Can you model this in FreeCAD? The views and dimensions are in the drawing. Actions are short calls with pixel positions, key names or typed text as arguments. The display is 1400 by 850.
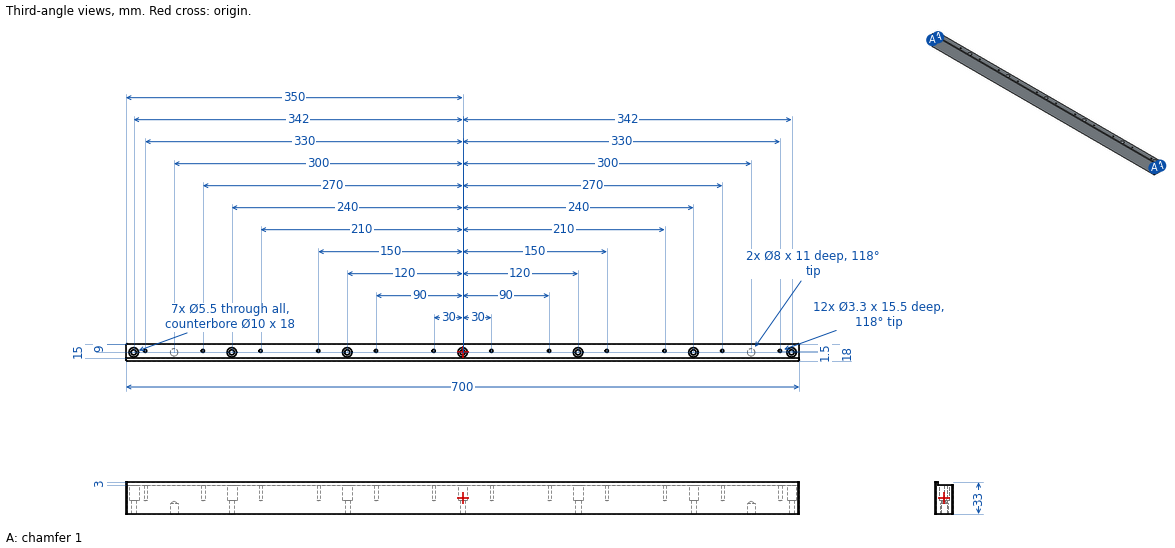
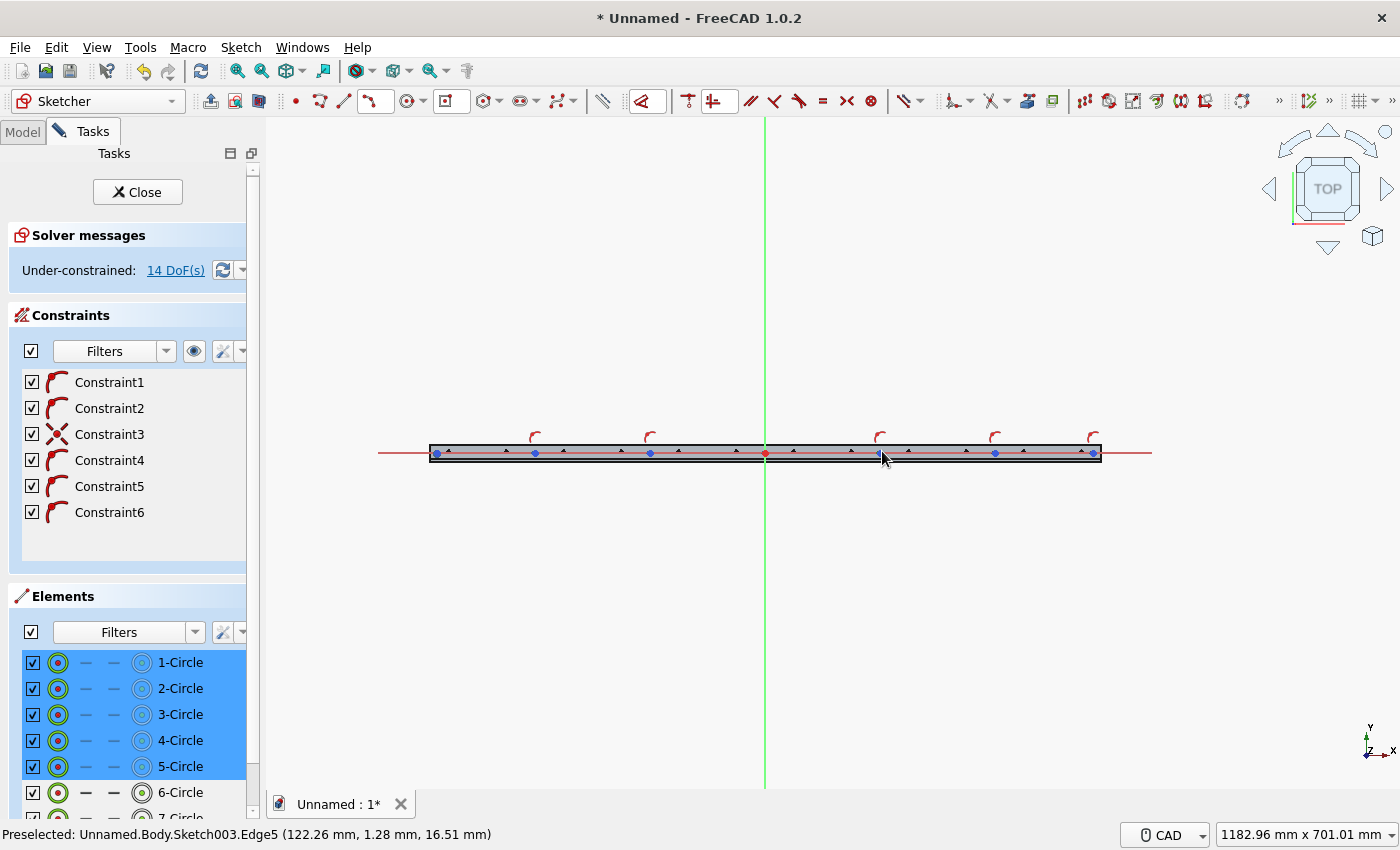
scroll(997, 451, up, 11)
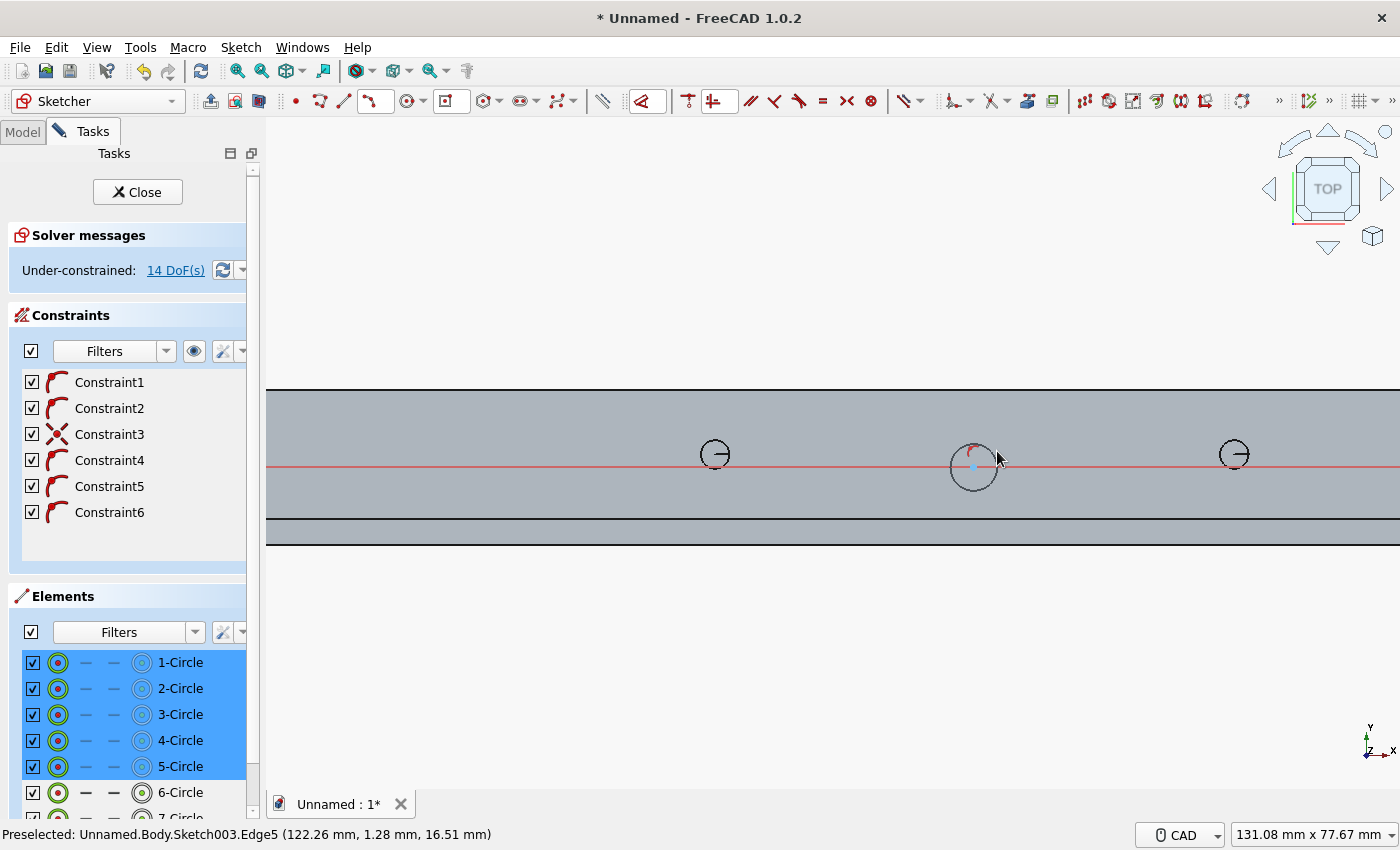
click(990, 451)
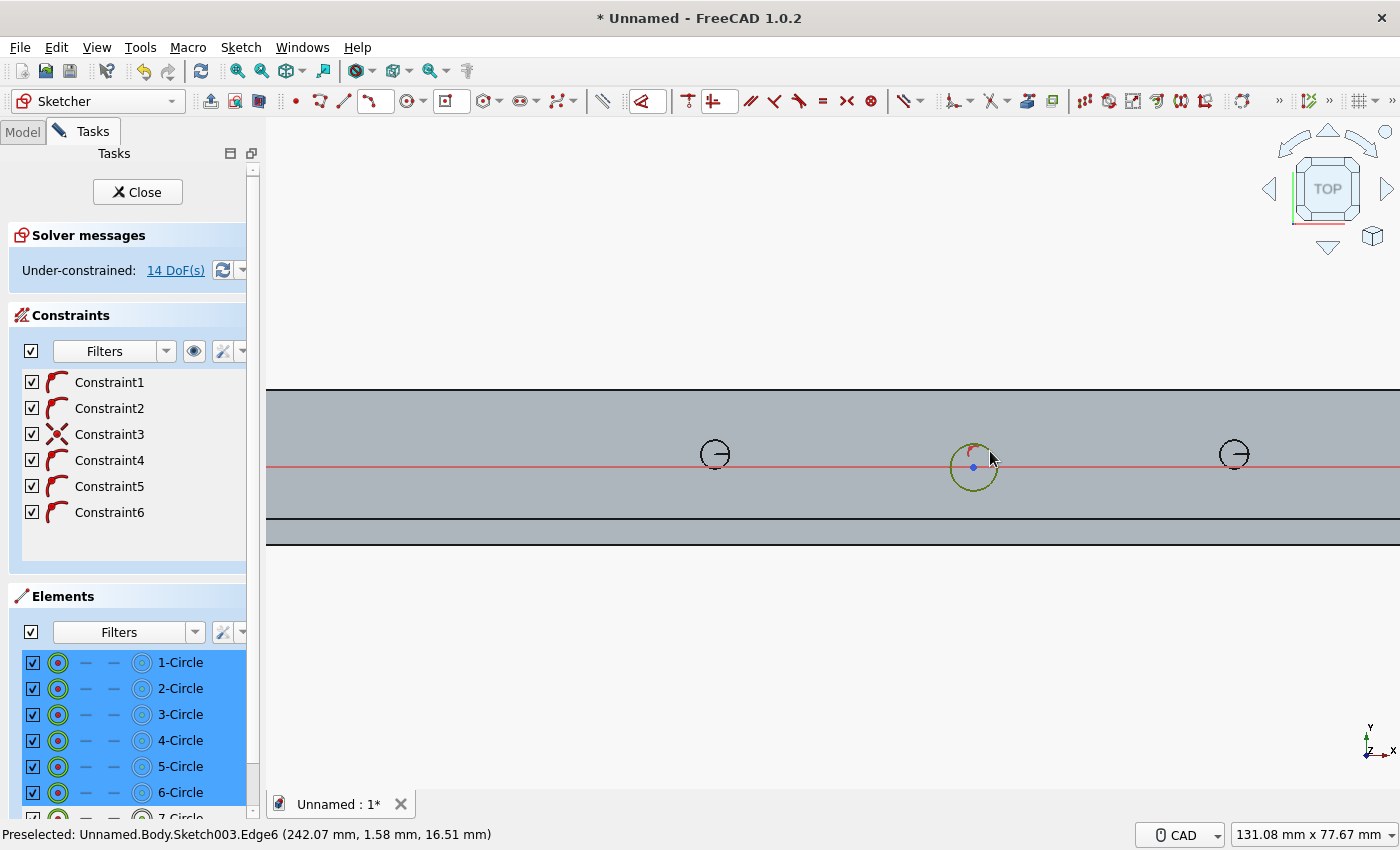
scroll(997, 451, down, 11)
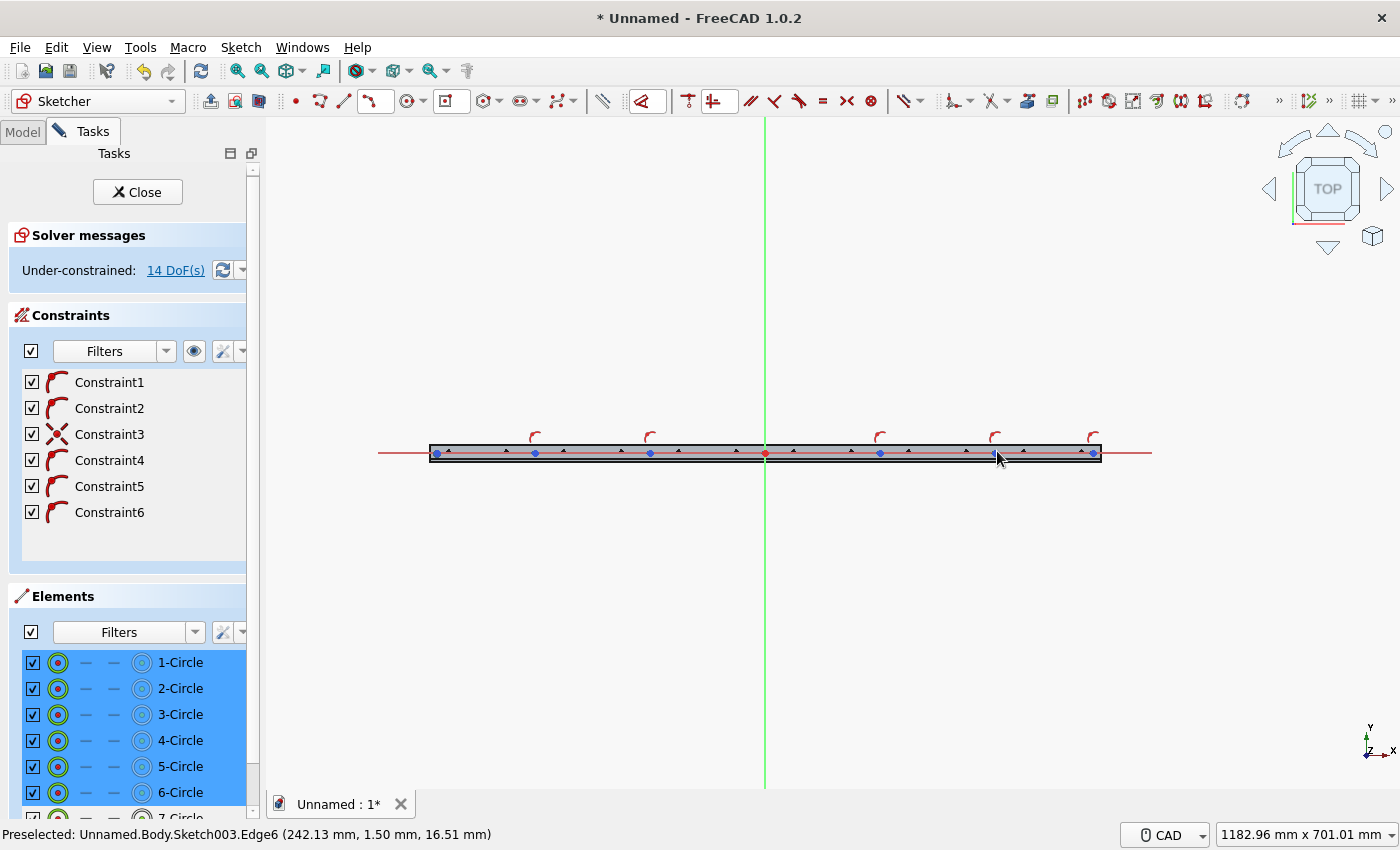
scroll(1095, 451, up, 11)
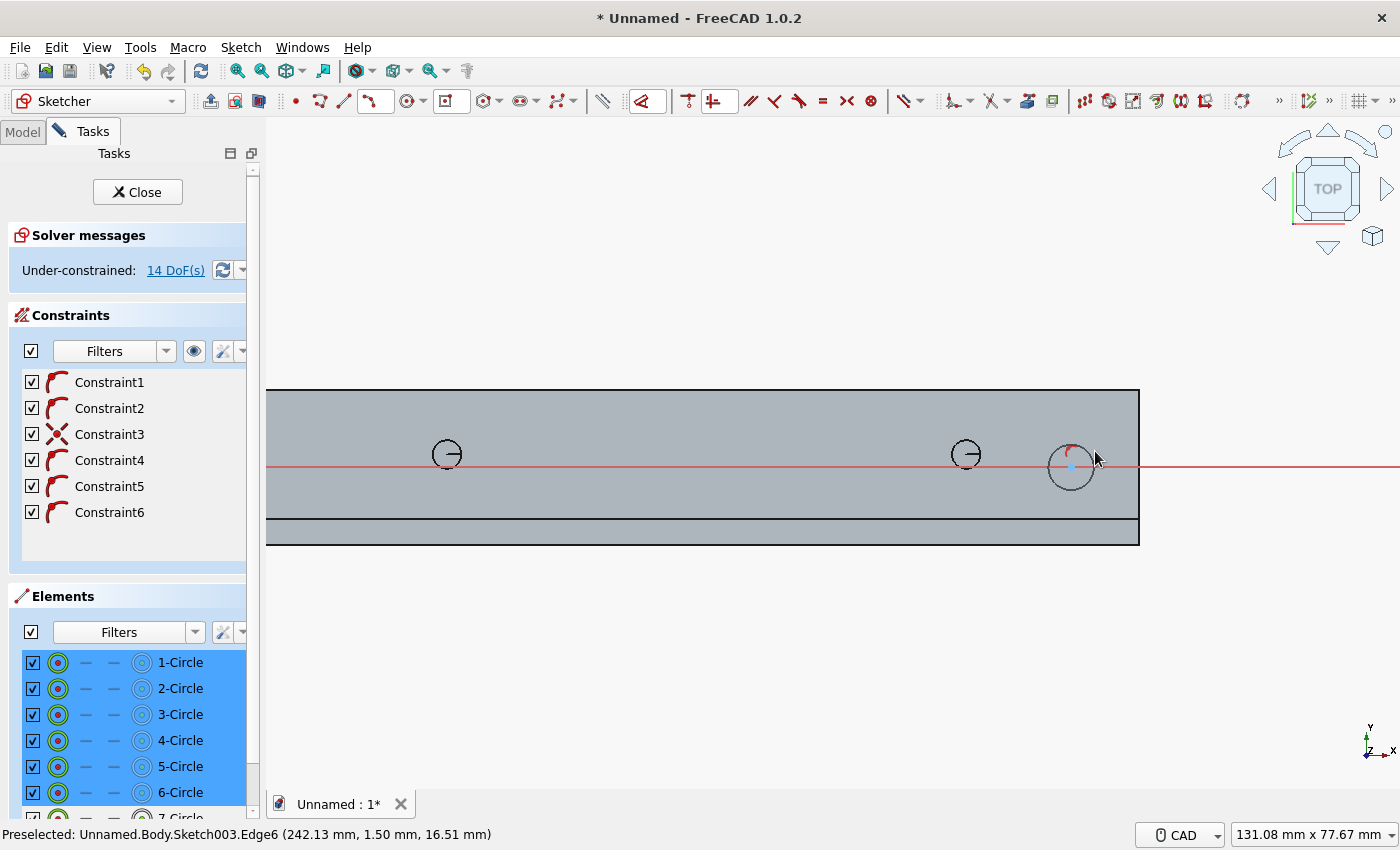
click(1087, 451)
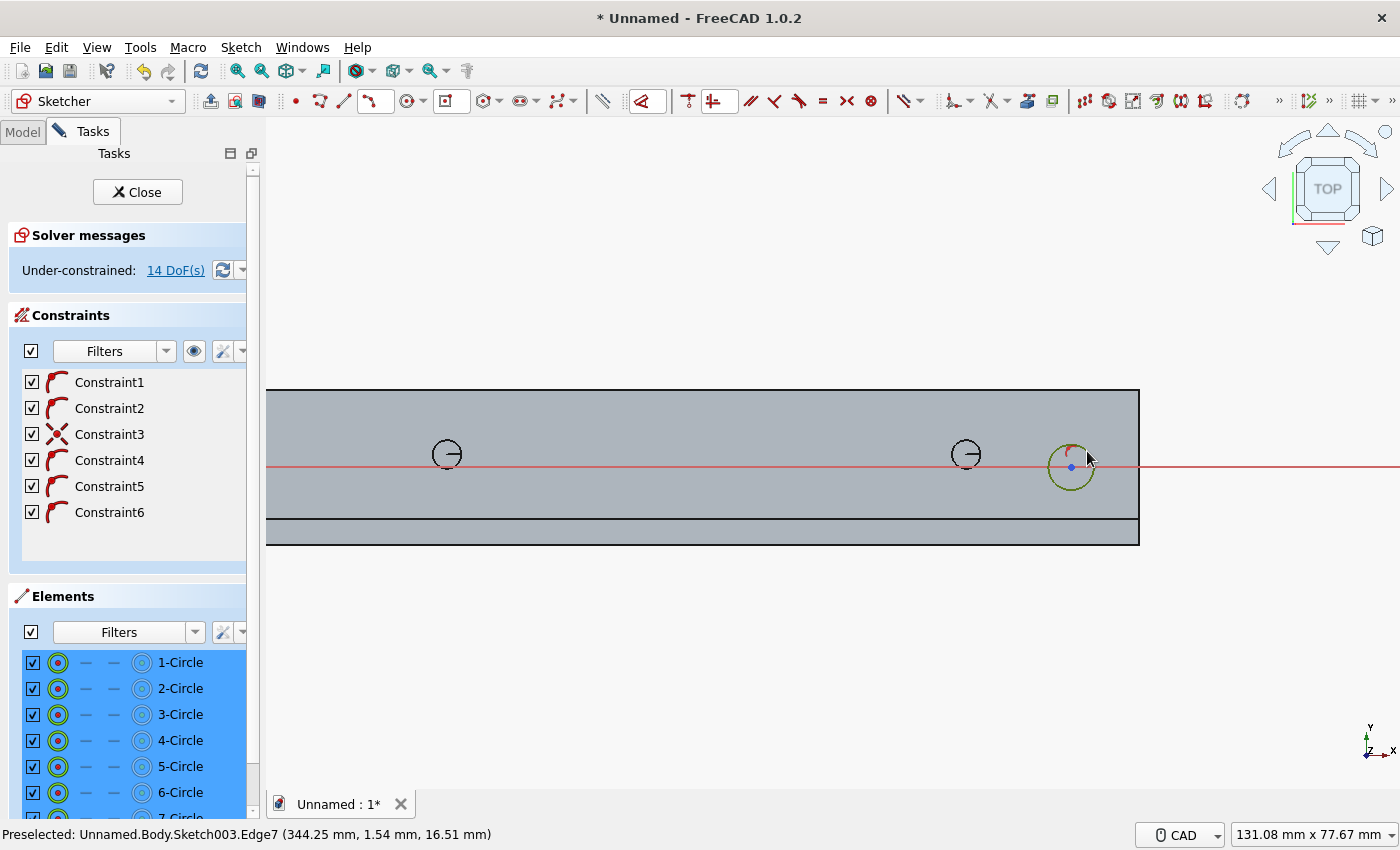
key(e)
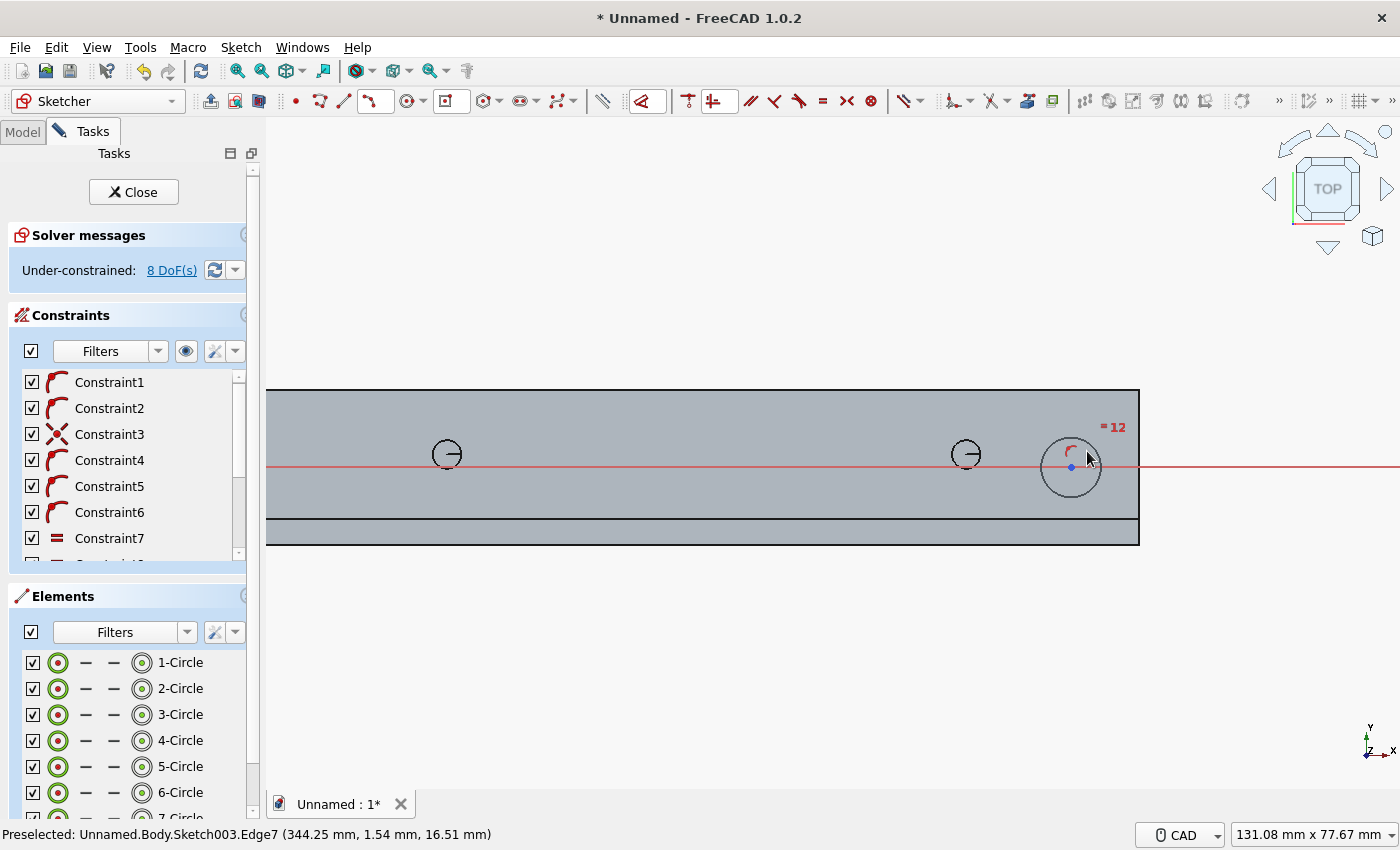
scroll(1095, 451, down, 11)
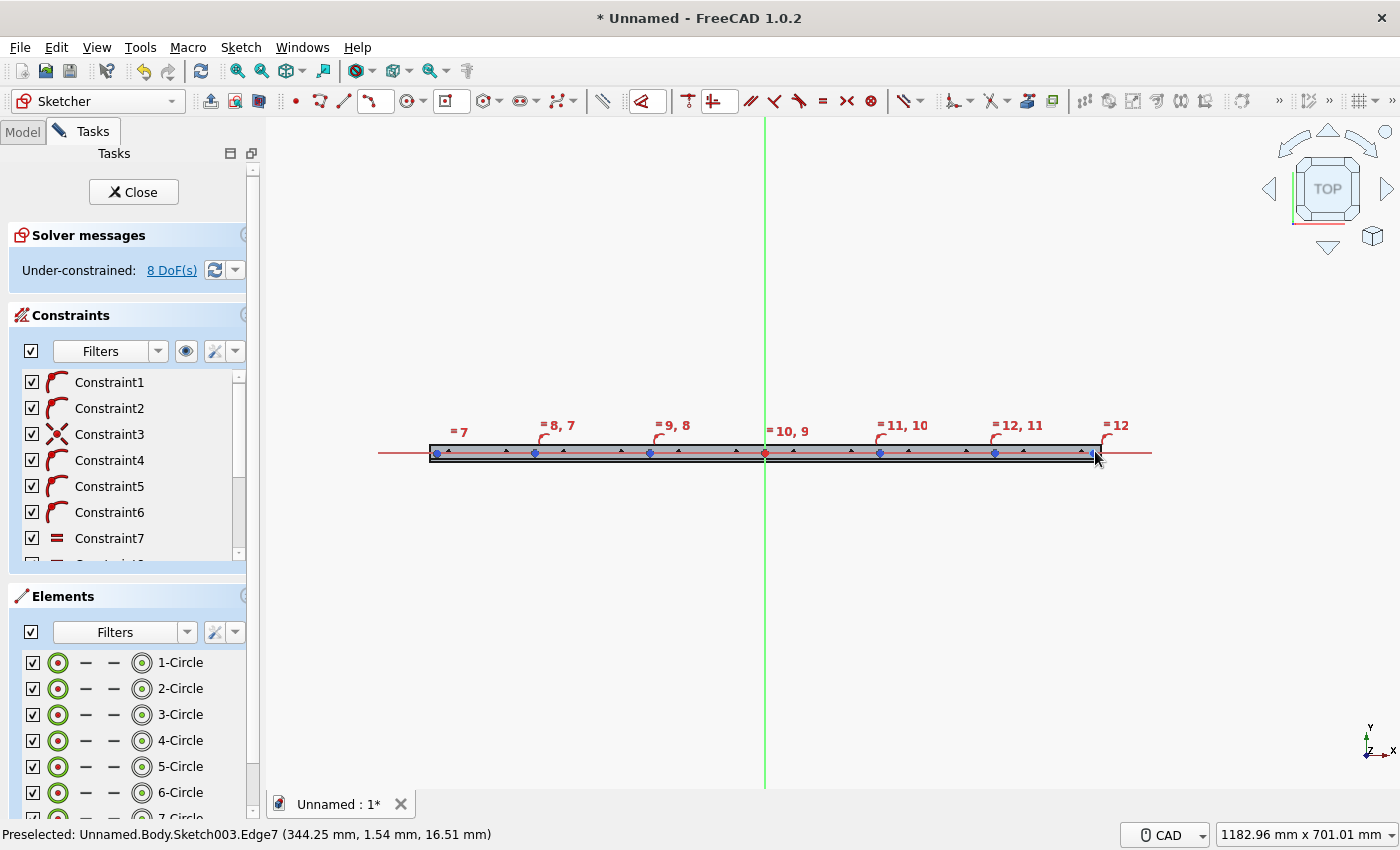
click(437, 454)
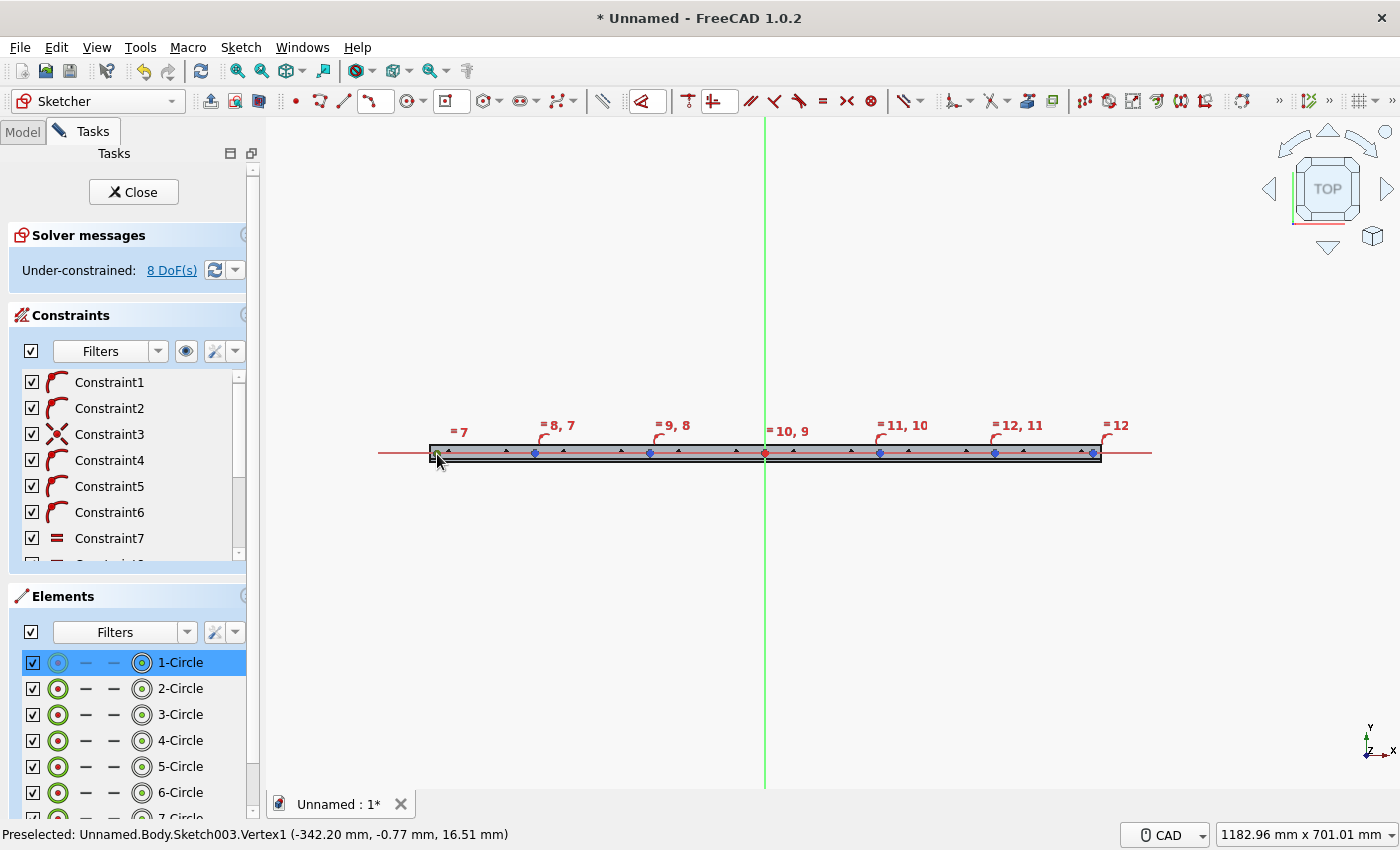
click(496, 453)